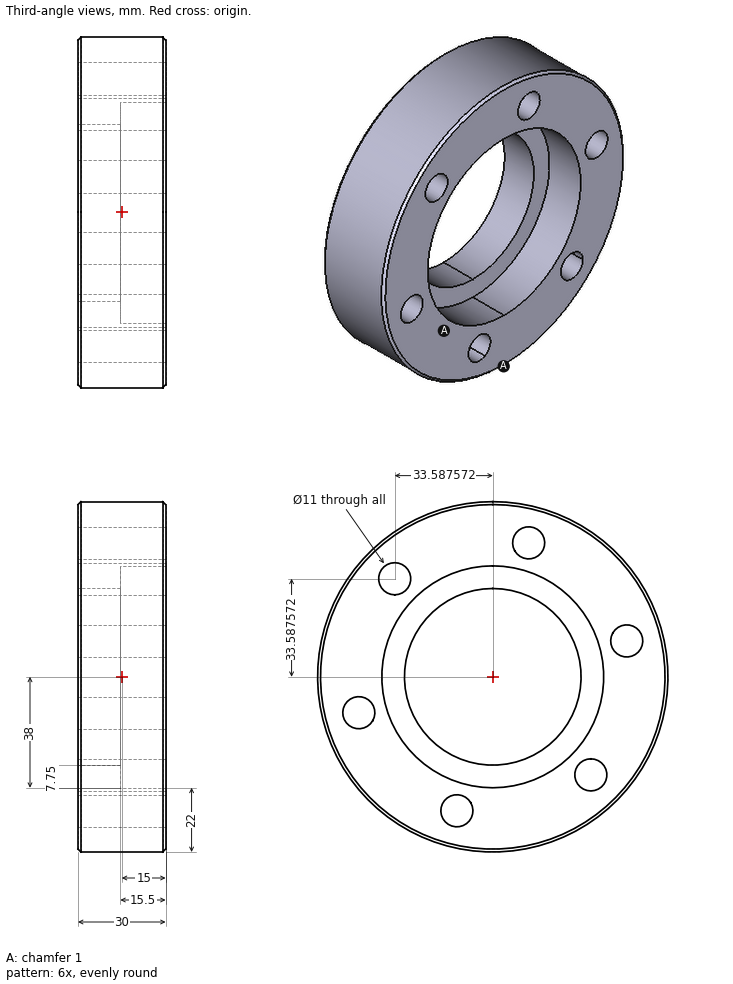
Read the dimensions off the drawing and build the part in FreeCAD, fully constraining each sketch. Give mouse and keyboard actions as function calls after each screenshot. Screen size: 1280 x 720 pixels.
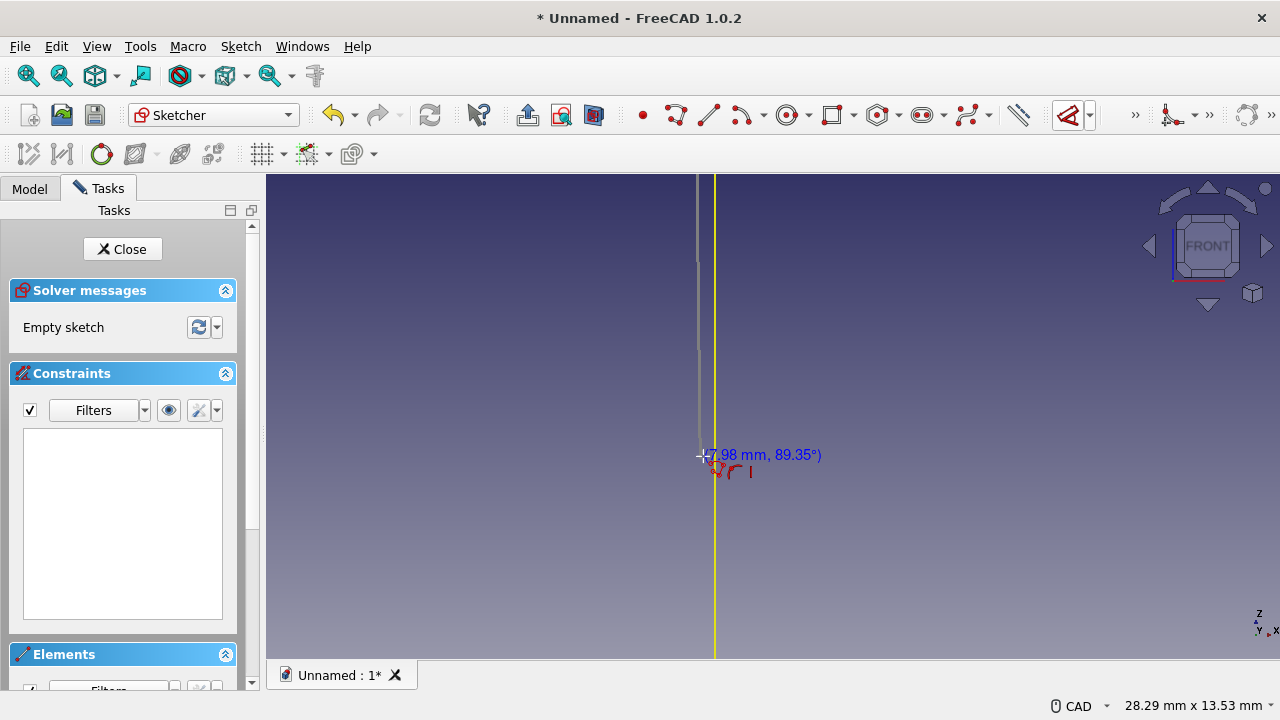
click(697, 451)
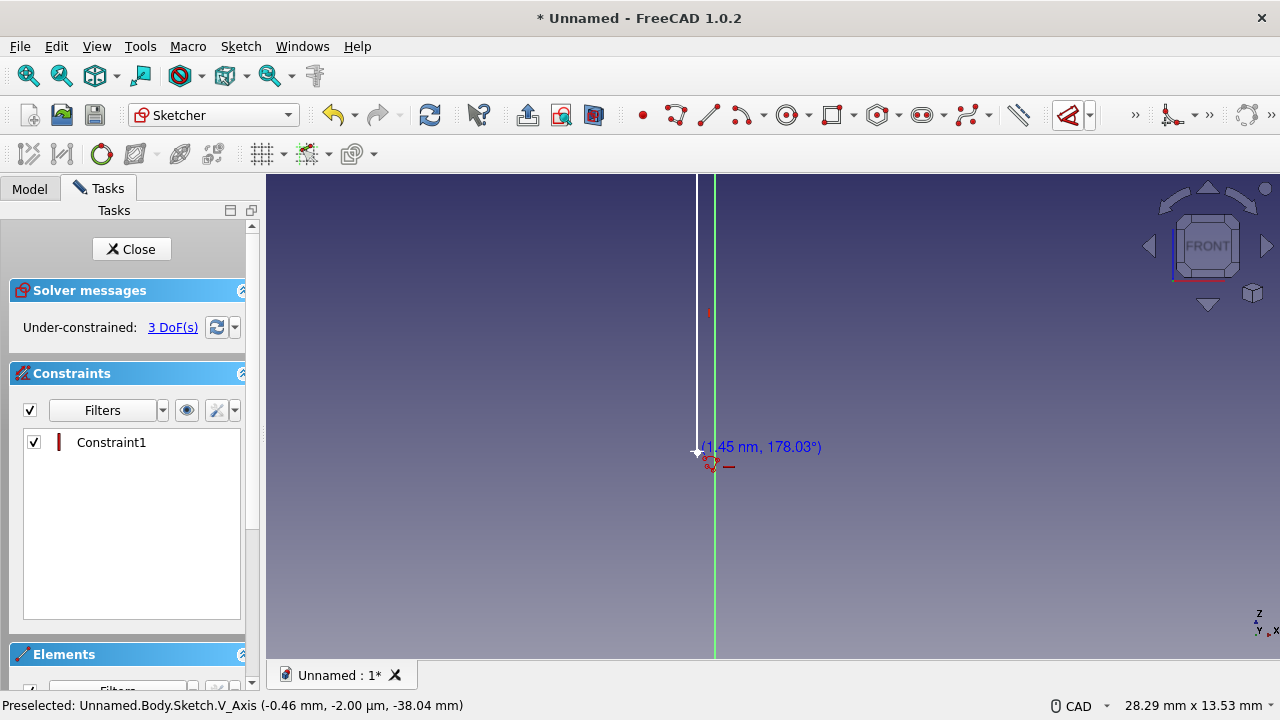
scroll(703, 456, down, 10)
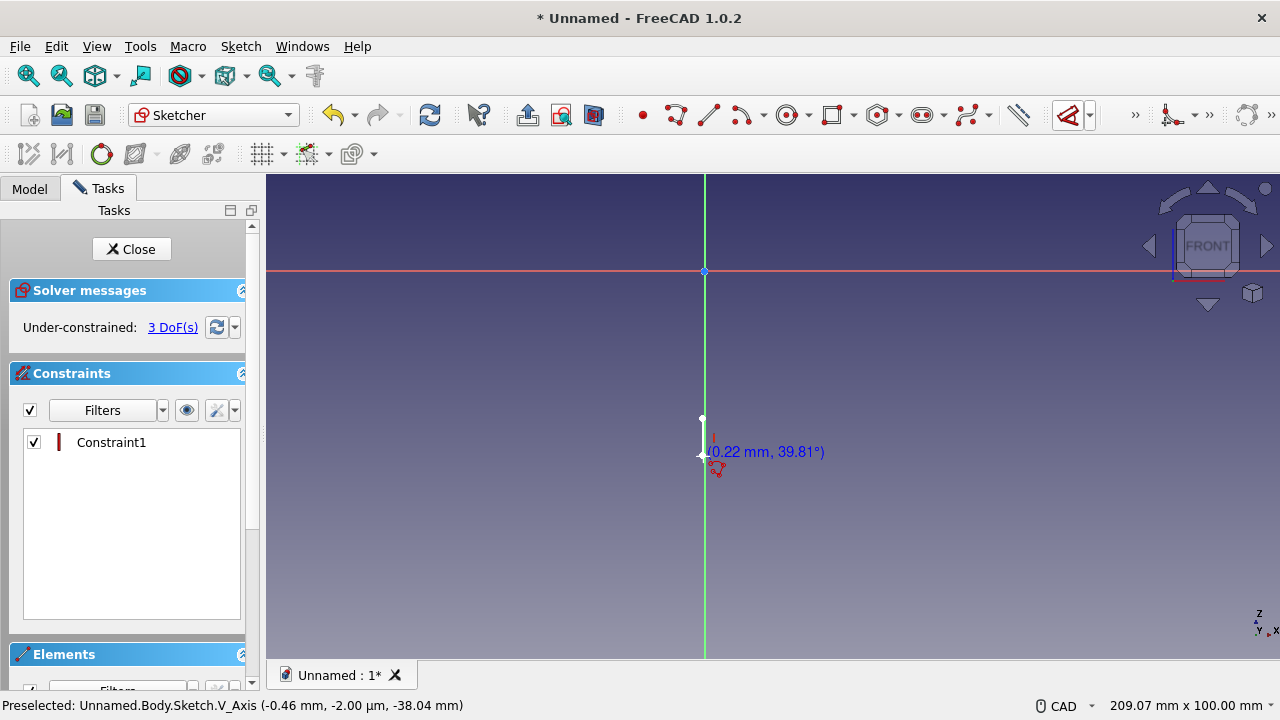
click(778, 456)
click(778, 562)
click(632, 562)
click(632, 418)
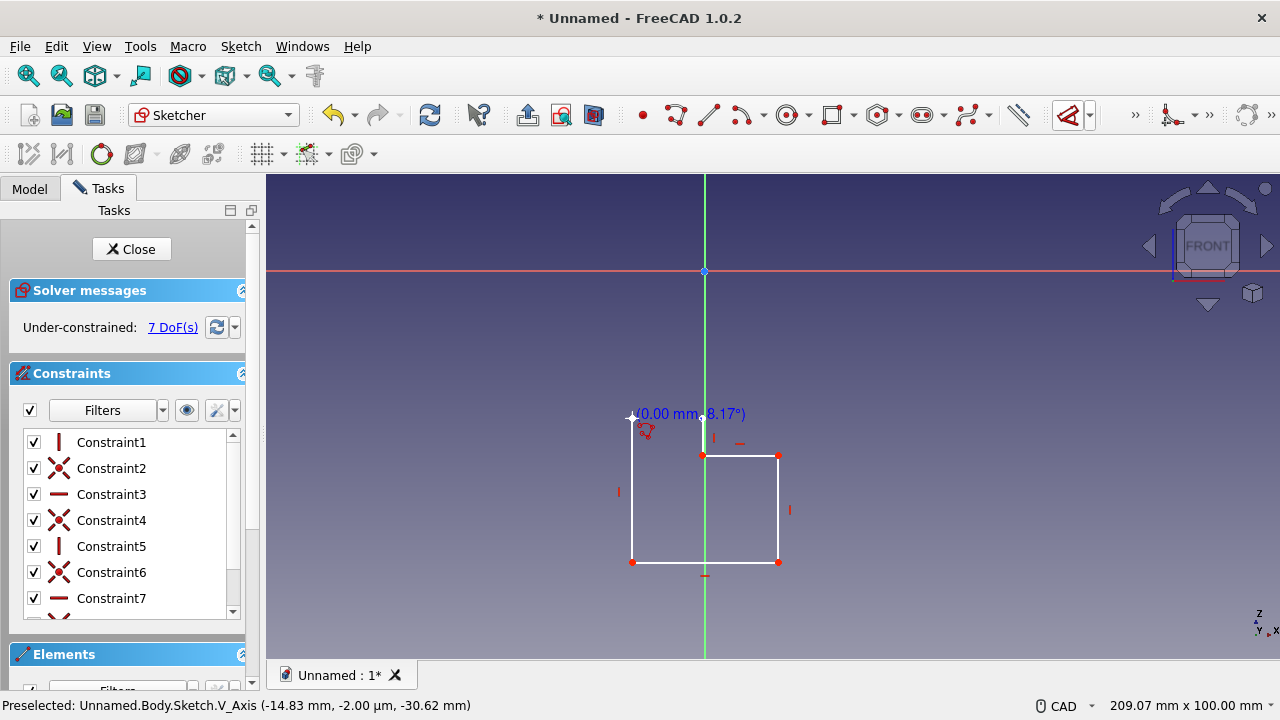
scroll(703, 418, up, 10)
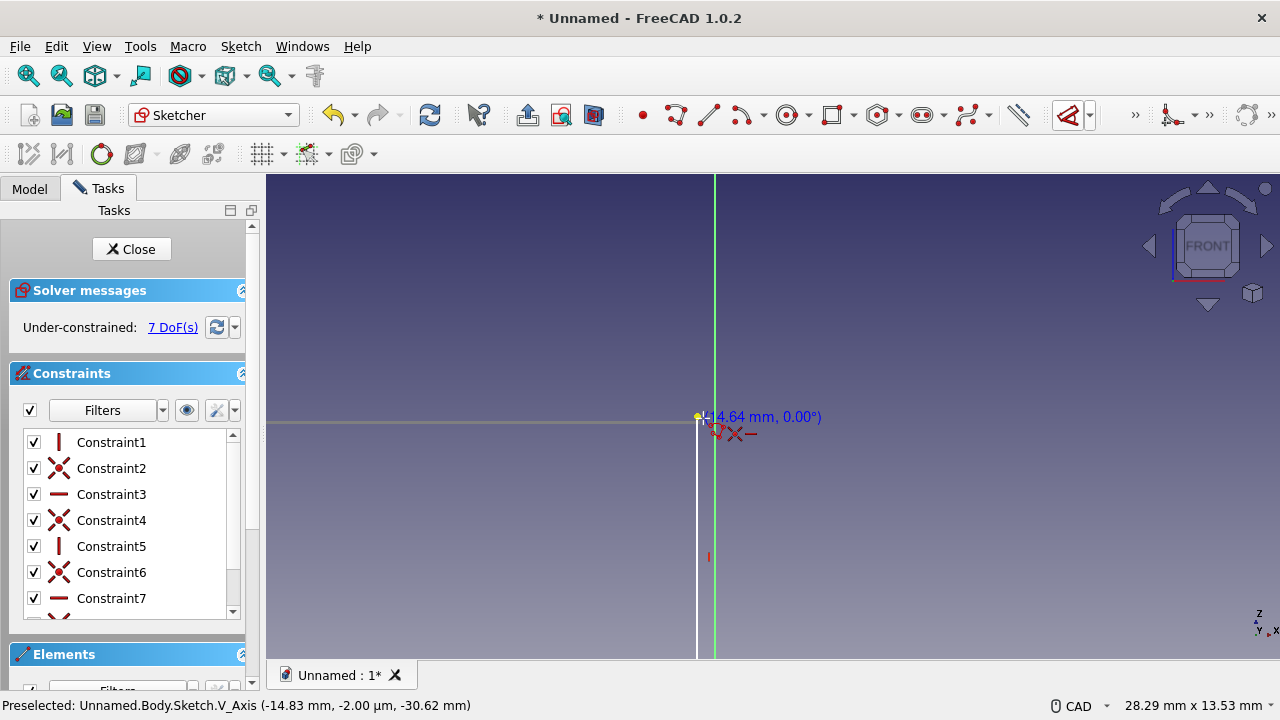
click(697, 417)
key(Escape)
key(Escape)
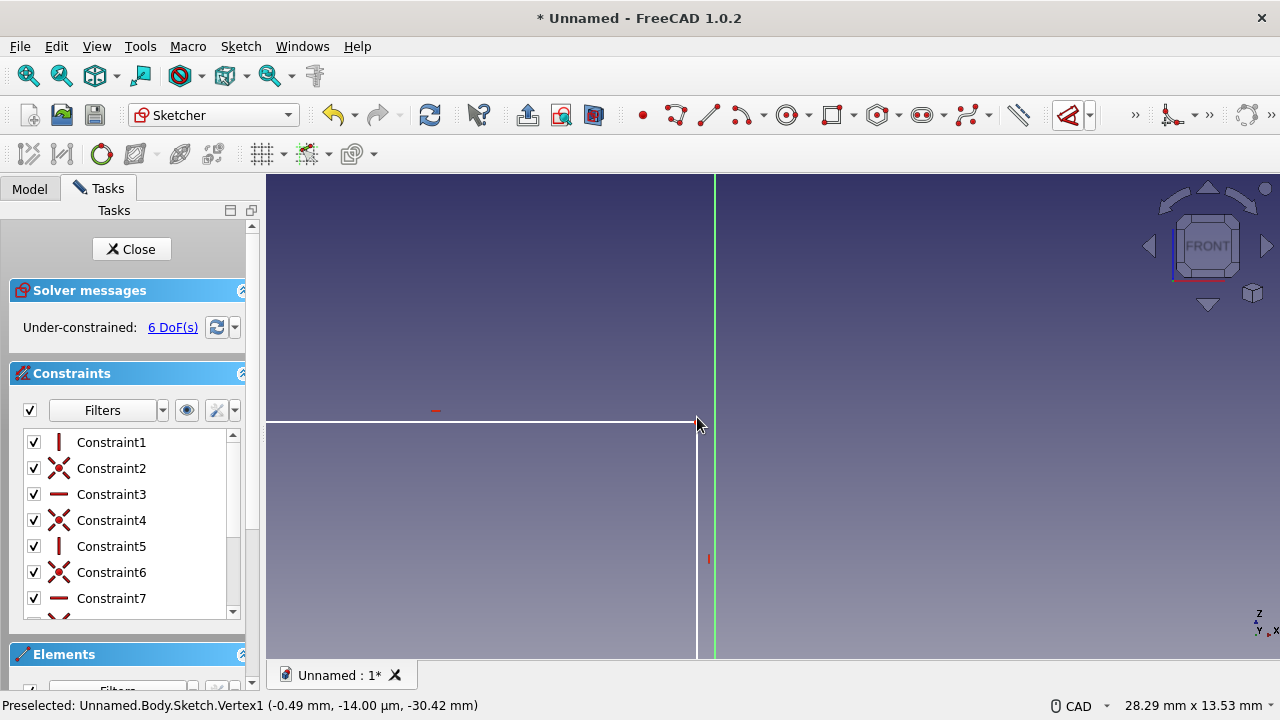
scroll(703, 418, down, 10)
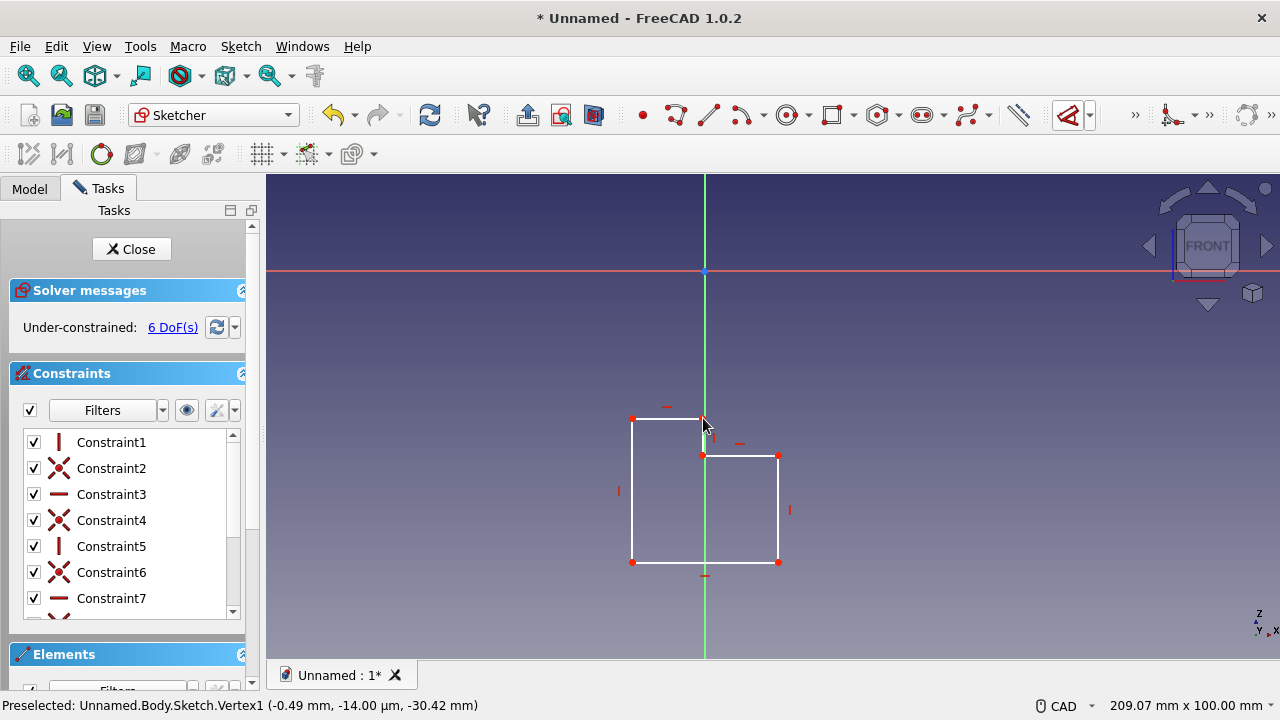
click(778, 488)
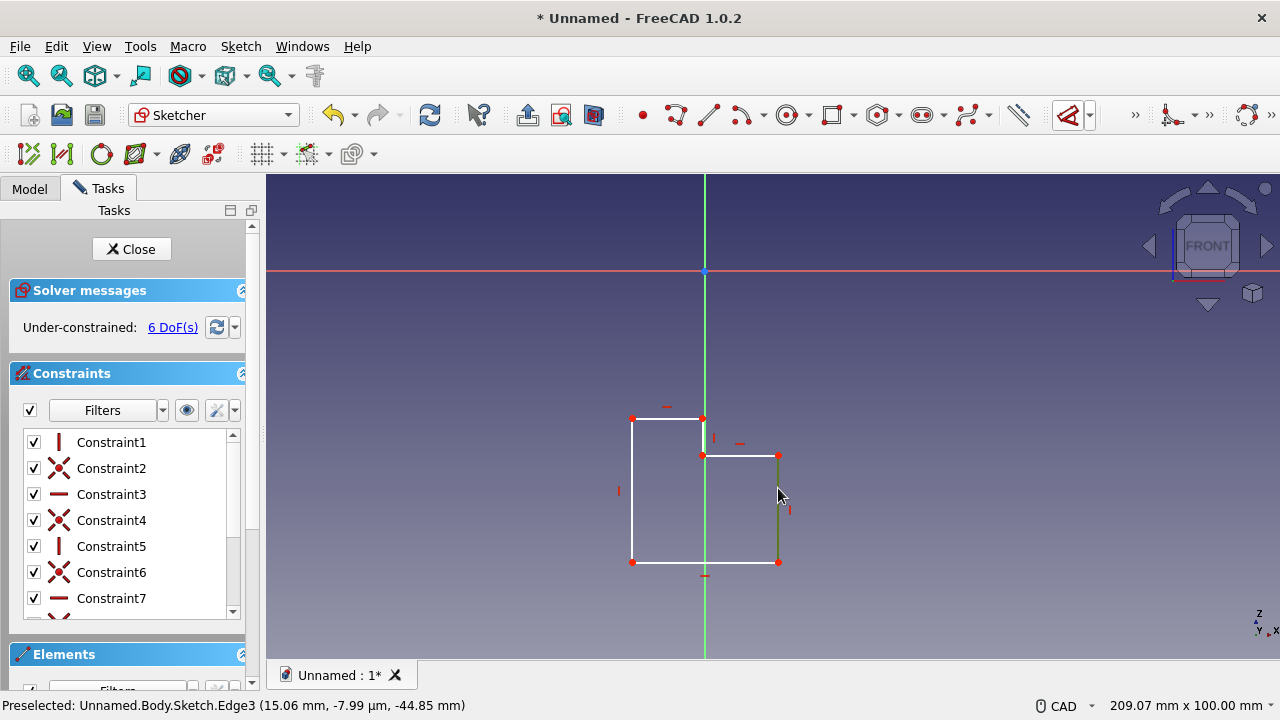
click(1090, 116)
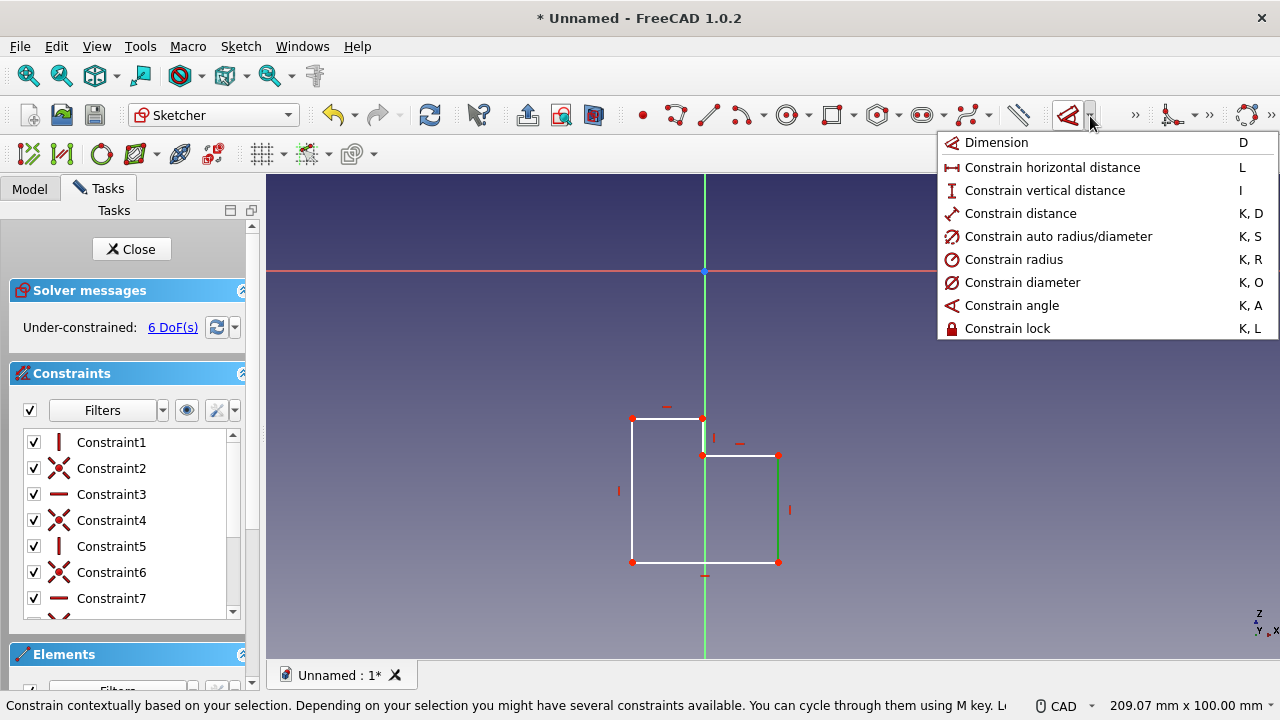
click(1108, 190)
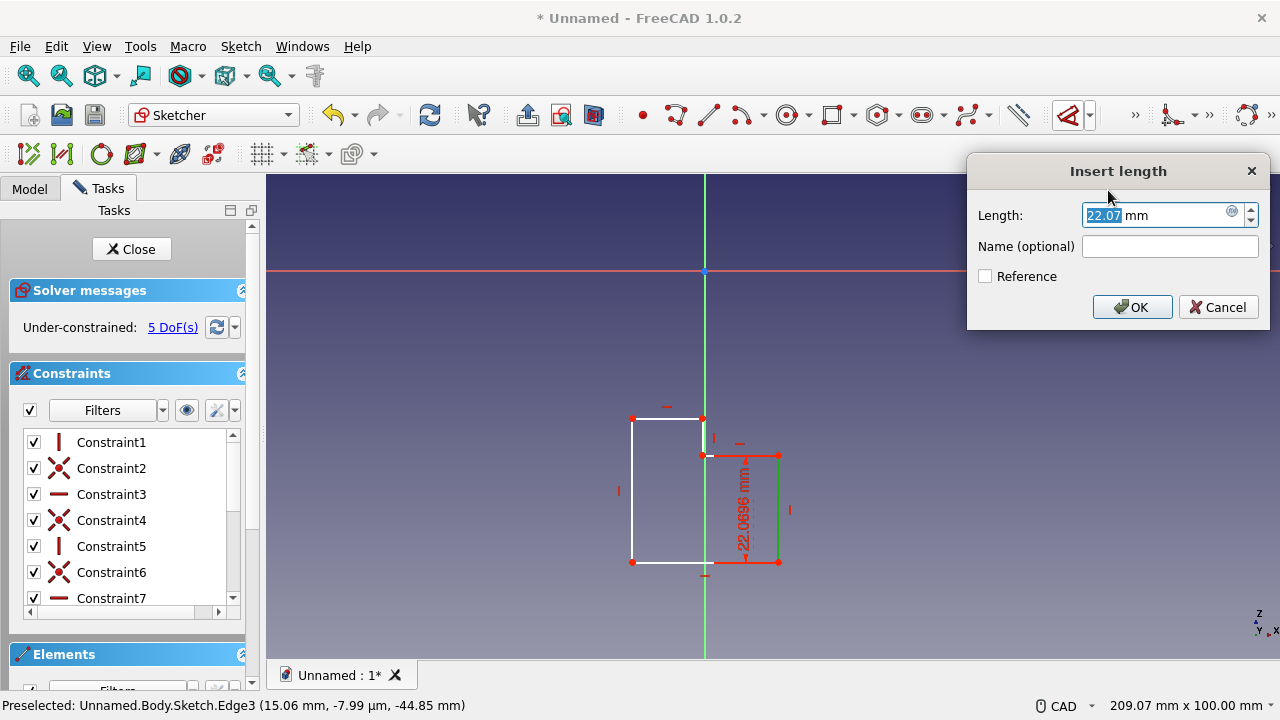
text(22)
key(Return)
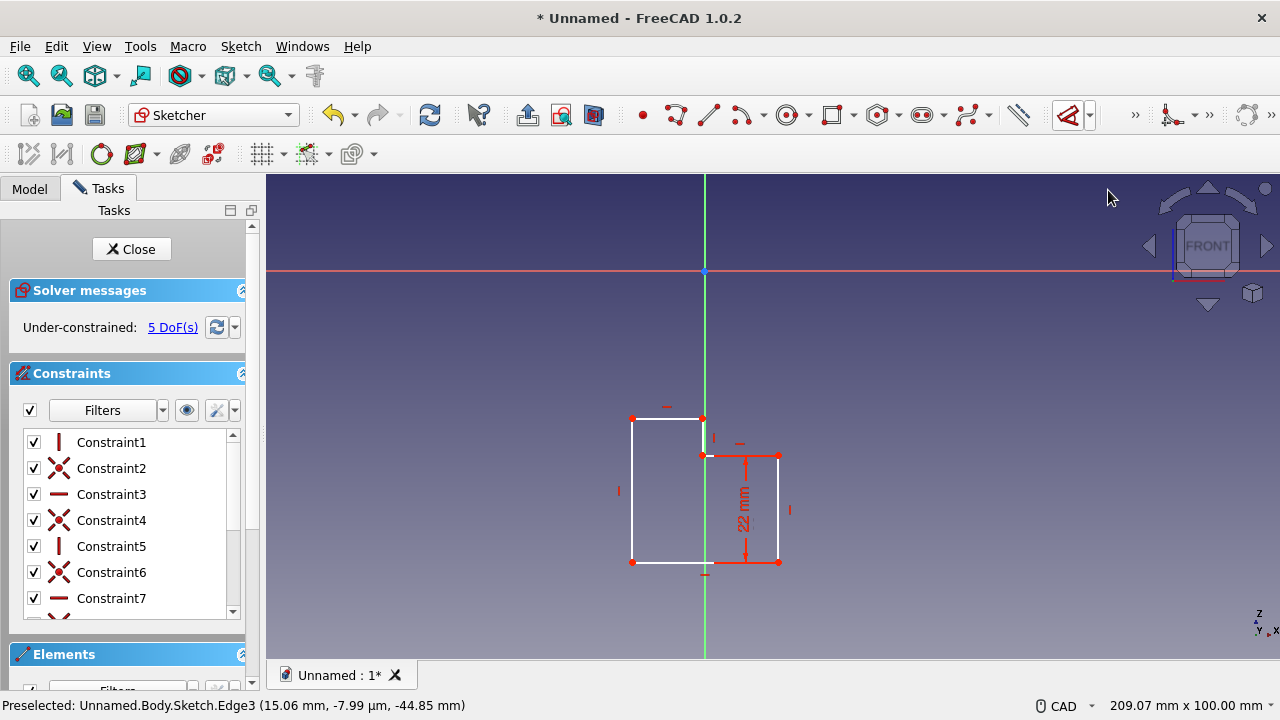
click(734, 563)